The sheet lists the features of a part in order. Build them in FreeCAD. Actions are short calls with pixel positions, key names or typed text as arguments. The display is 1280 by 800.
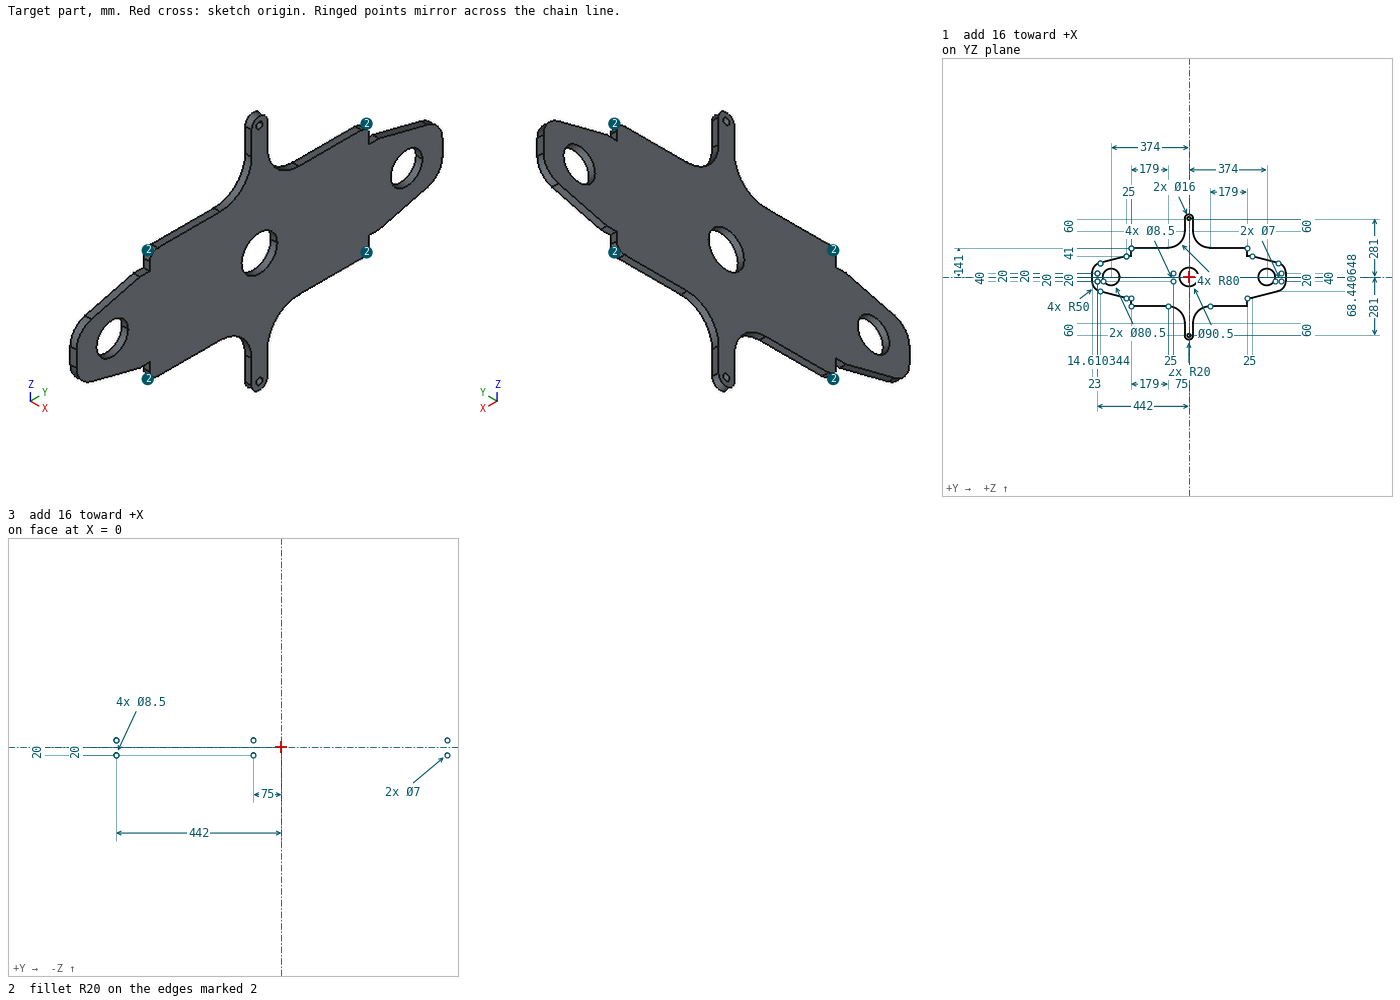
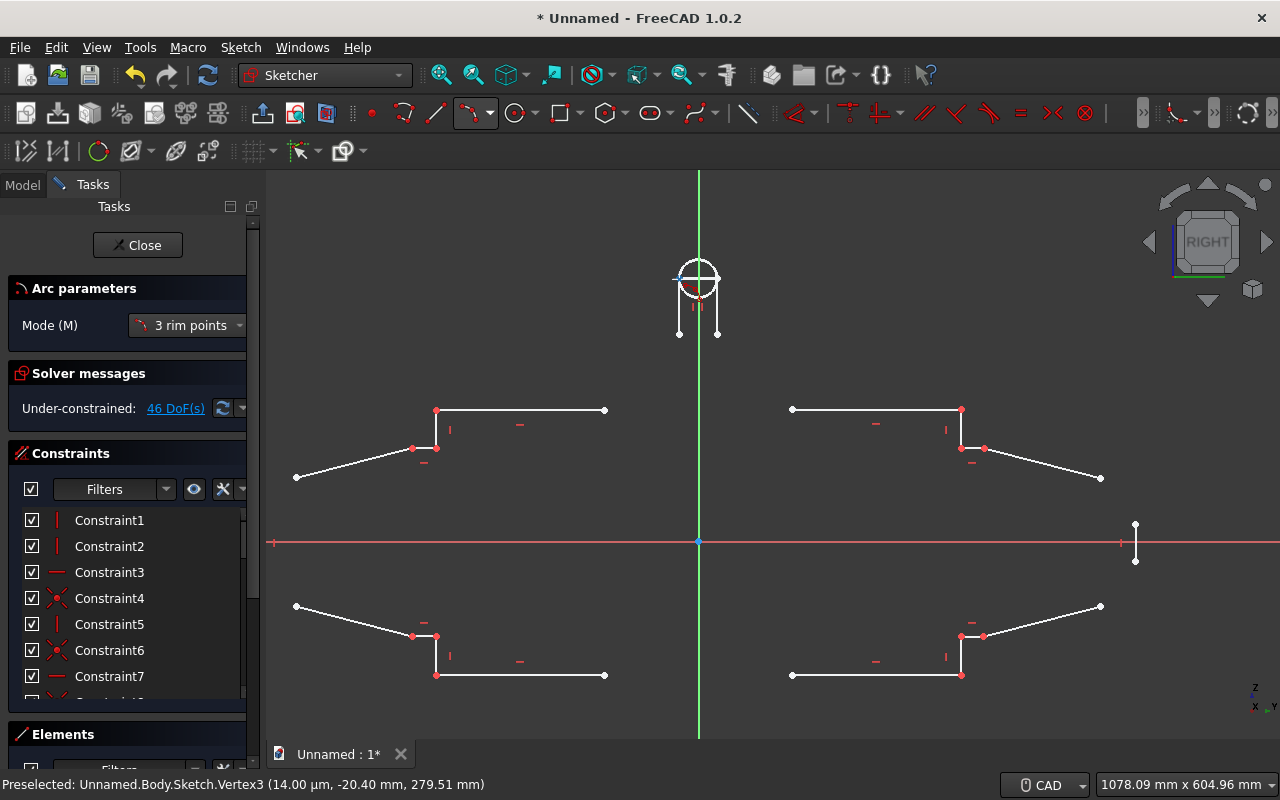
scroll(710, 262, up, 2)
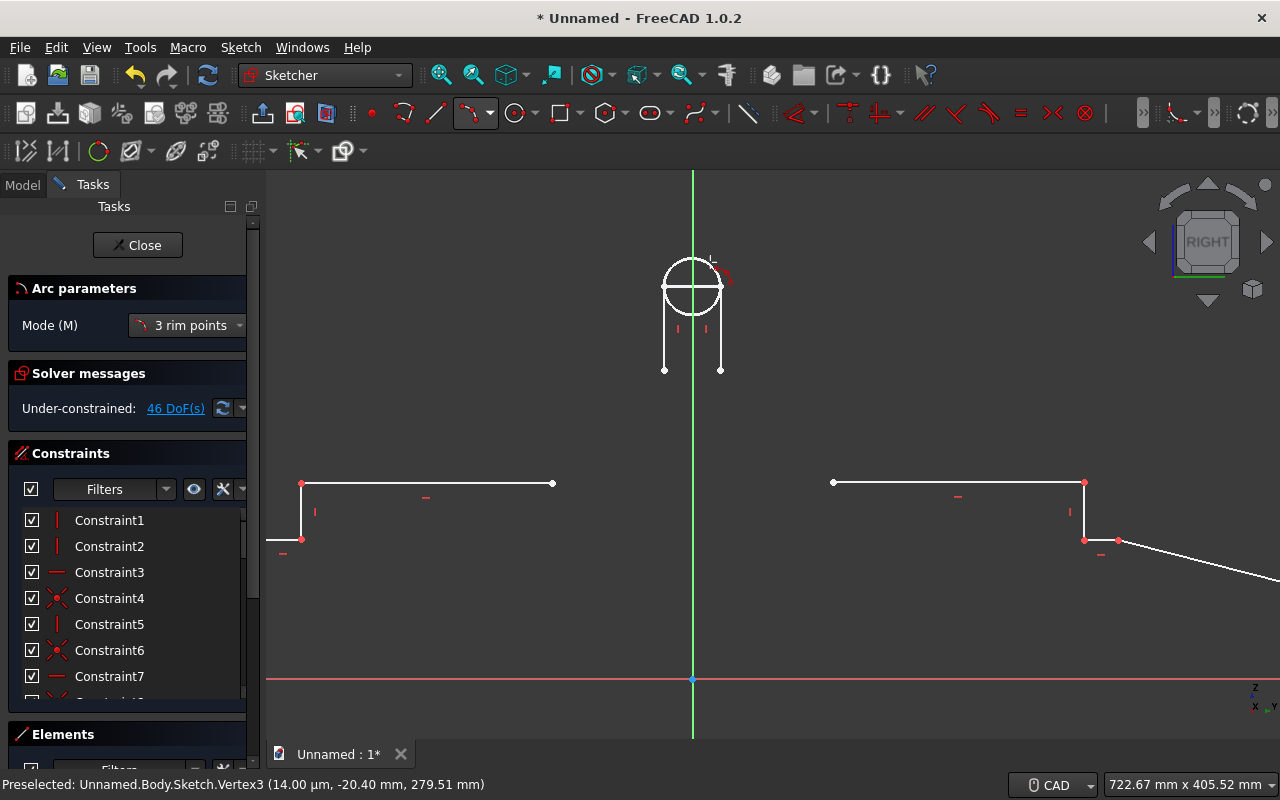
click(709, 262)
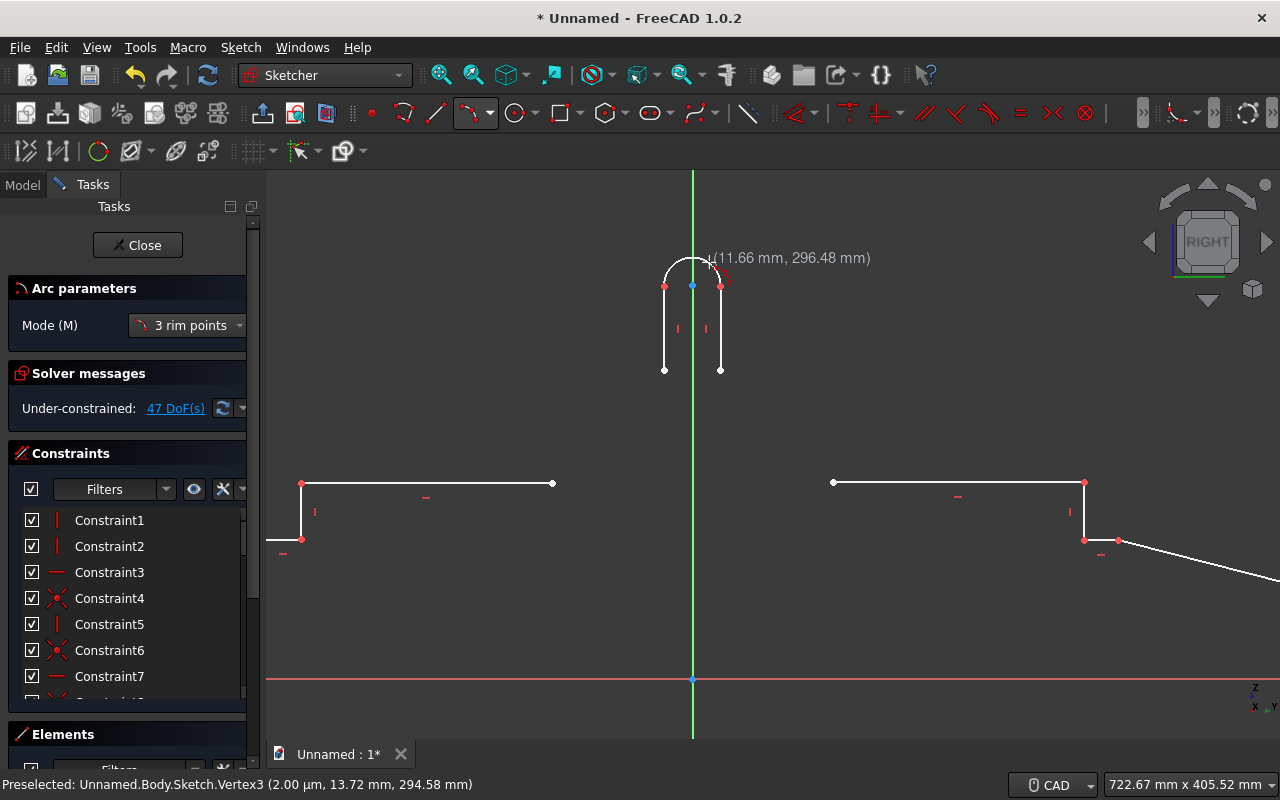
click(664, 370)
click(553, 483)
click(632, 448)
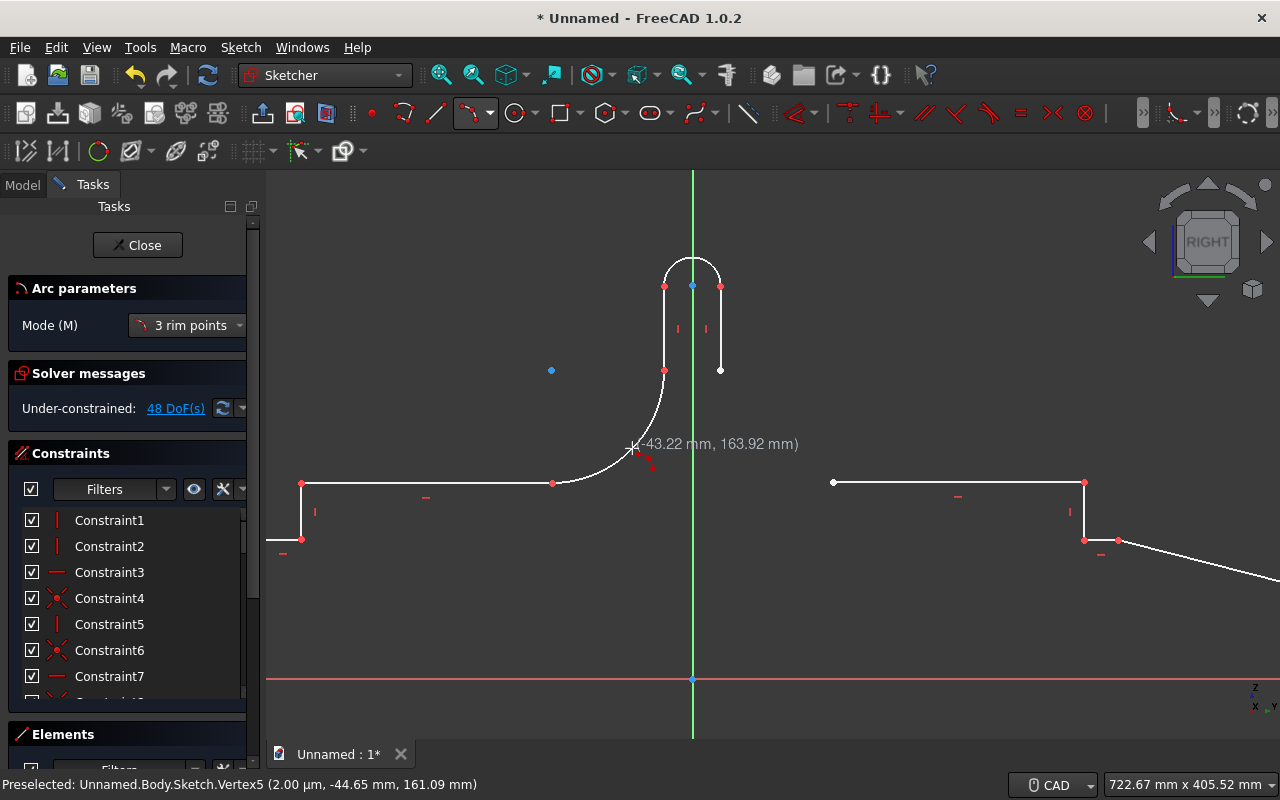
scroll(714, 271, down, 4)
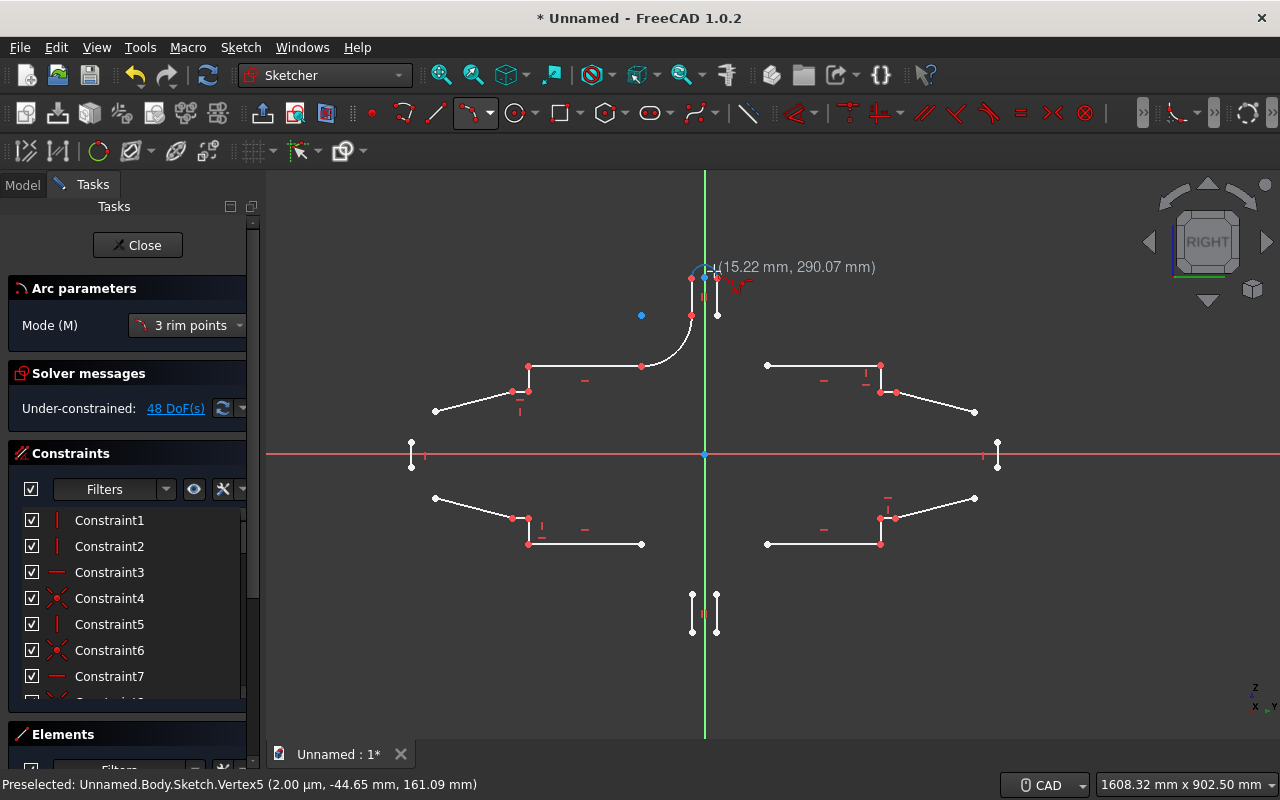
click(435, 412)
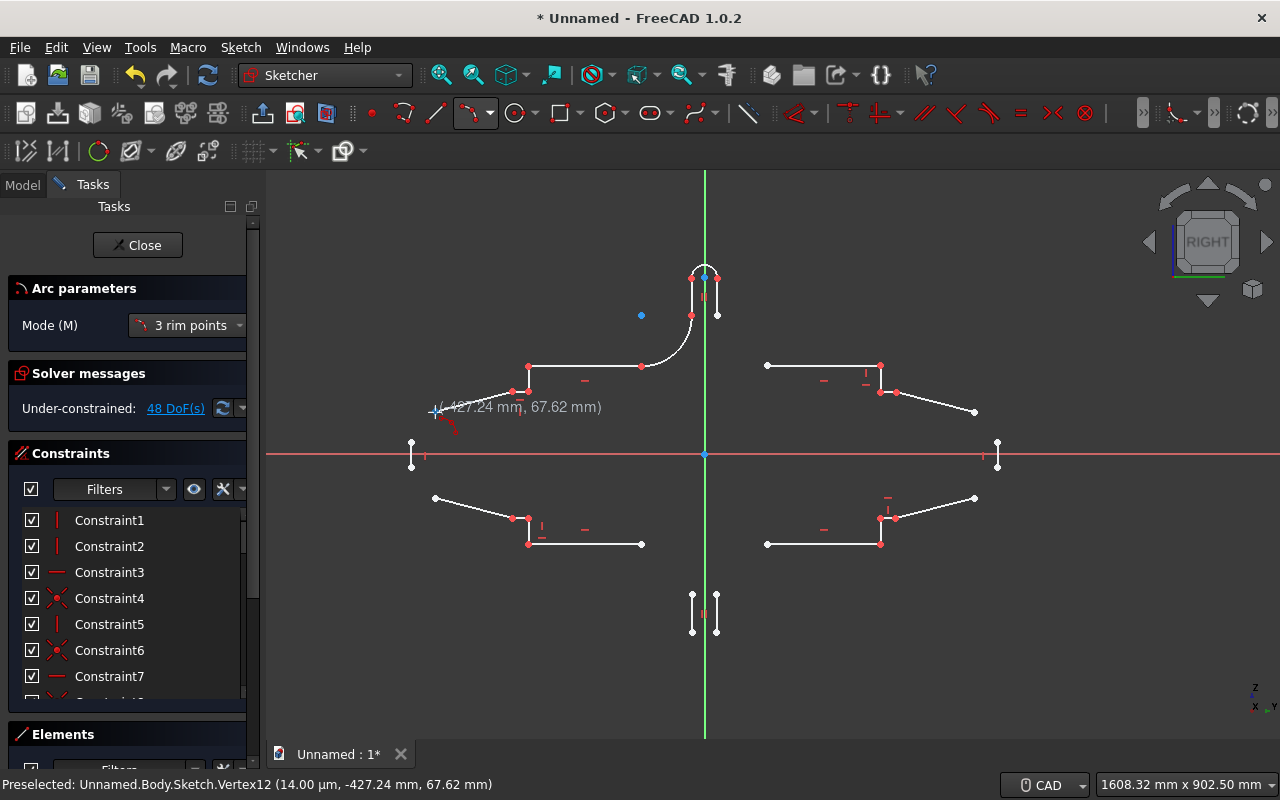
scroll(411, 442, up, 2)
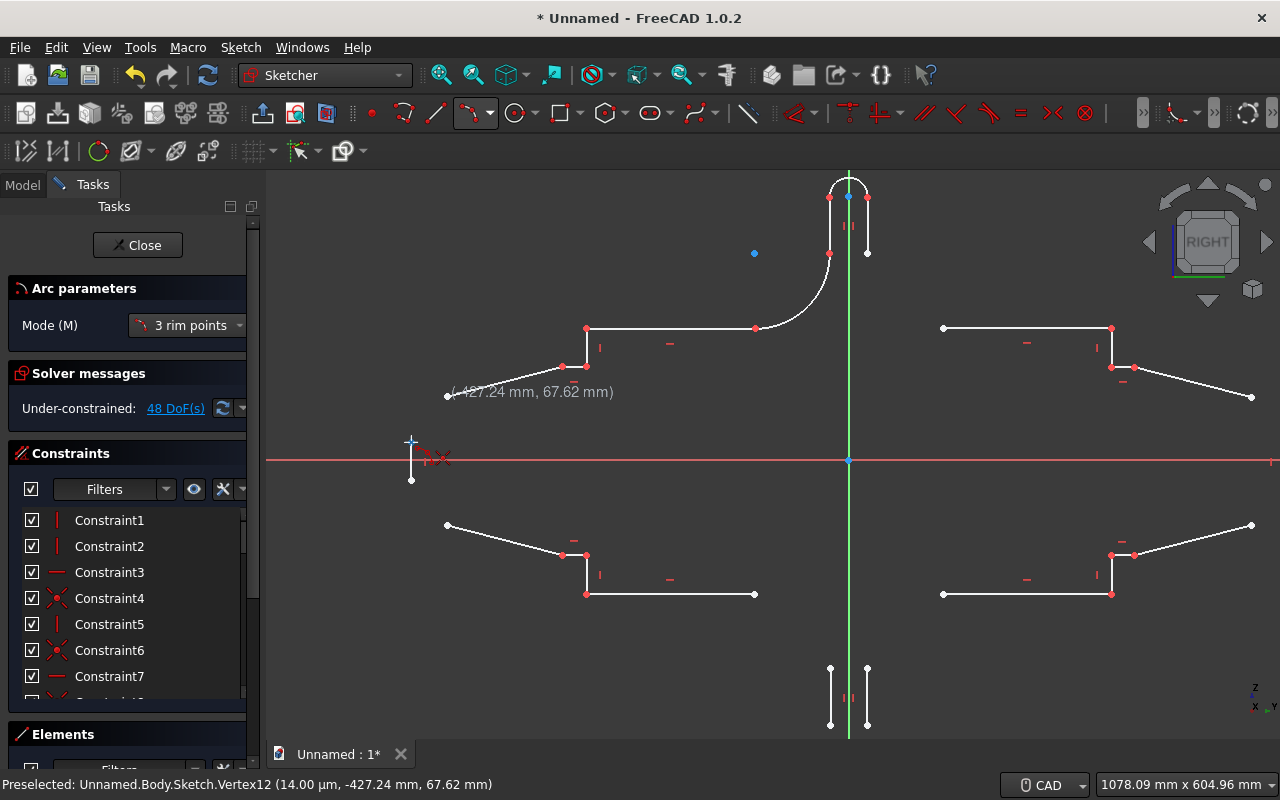
click(411, 443)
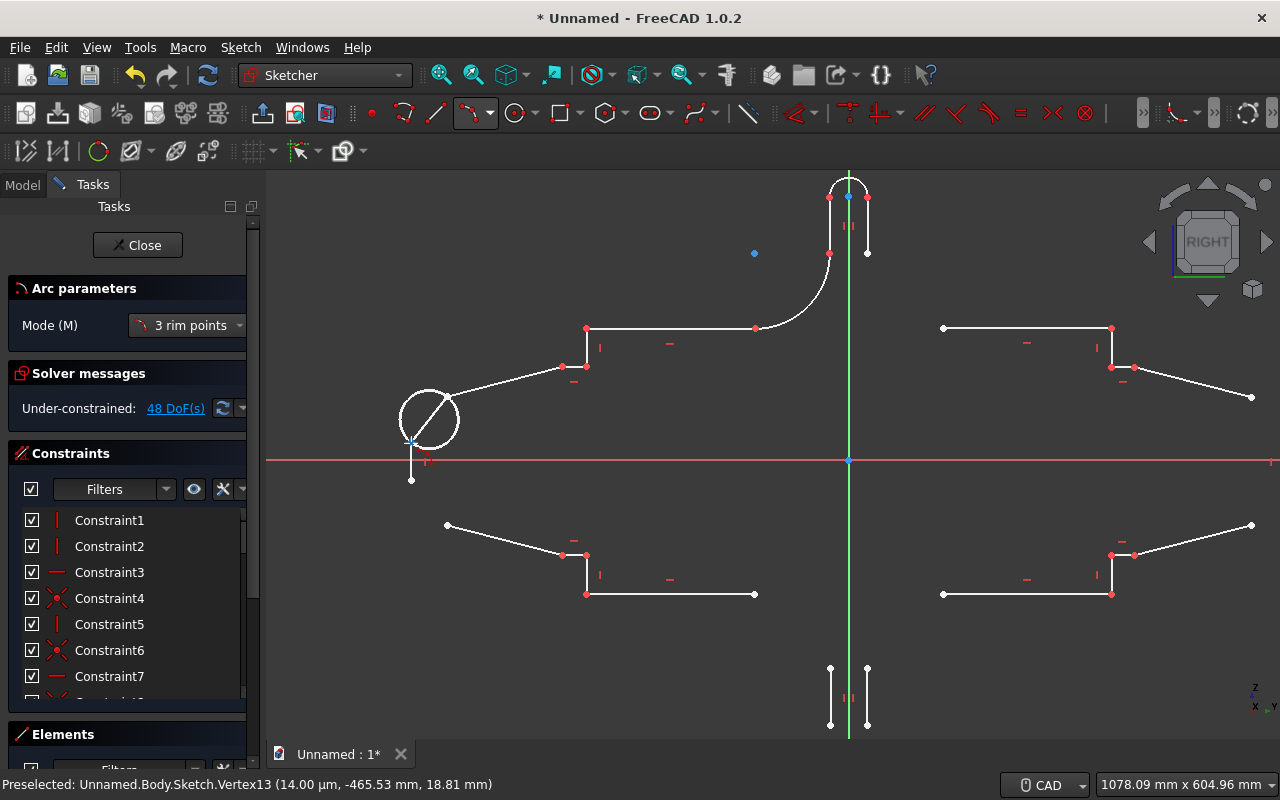
scroll(422, 413, up, 3)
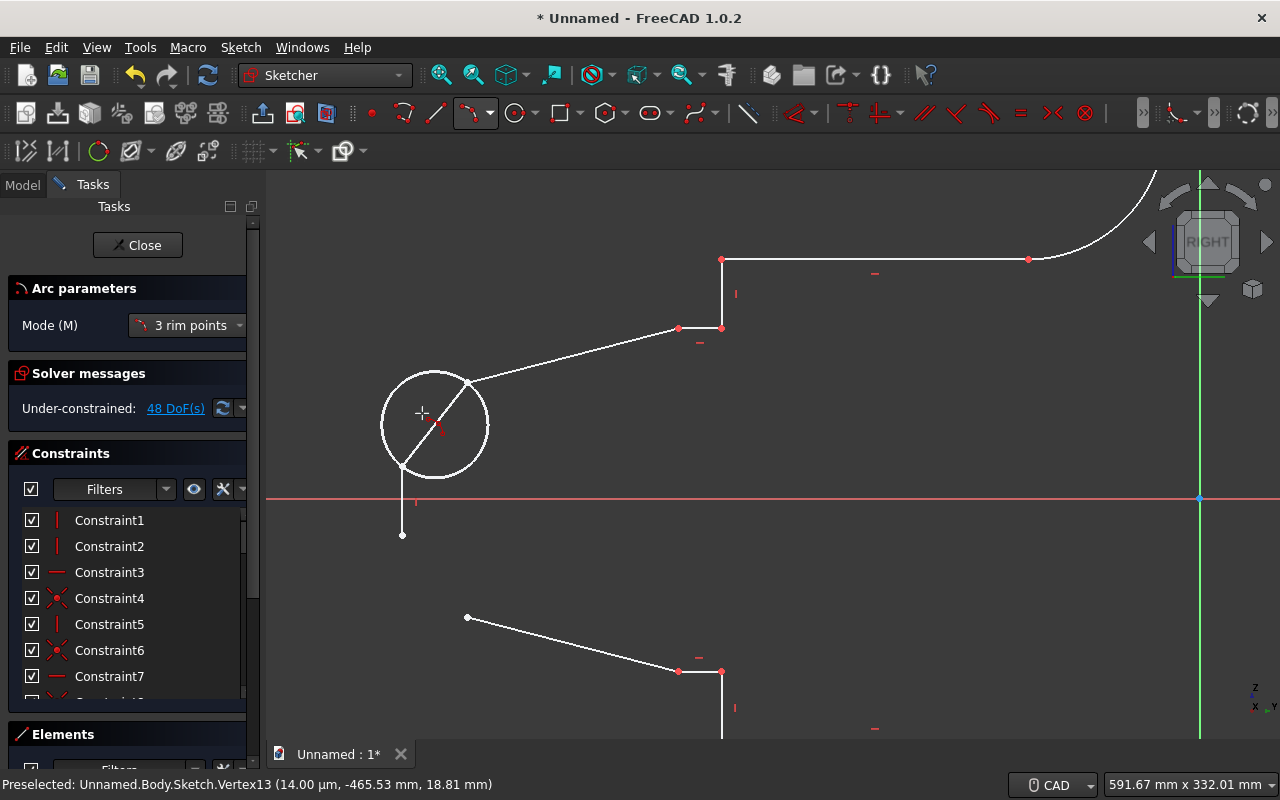
click(421, 412)